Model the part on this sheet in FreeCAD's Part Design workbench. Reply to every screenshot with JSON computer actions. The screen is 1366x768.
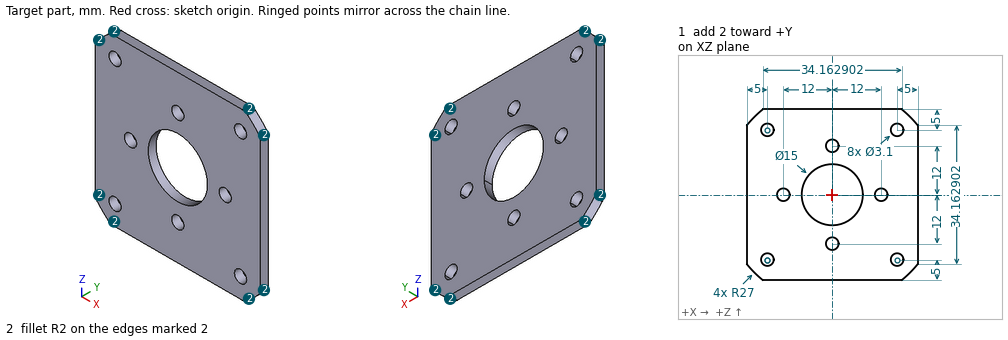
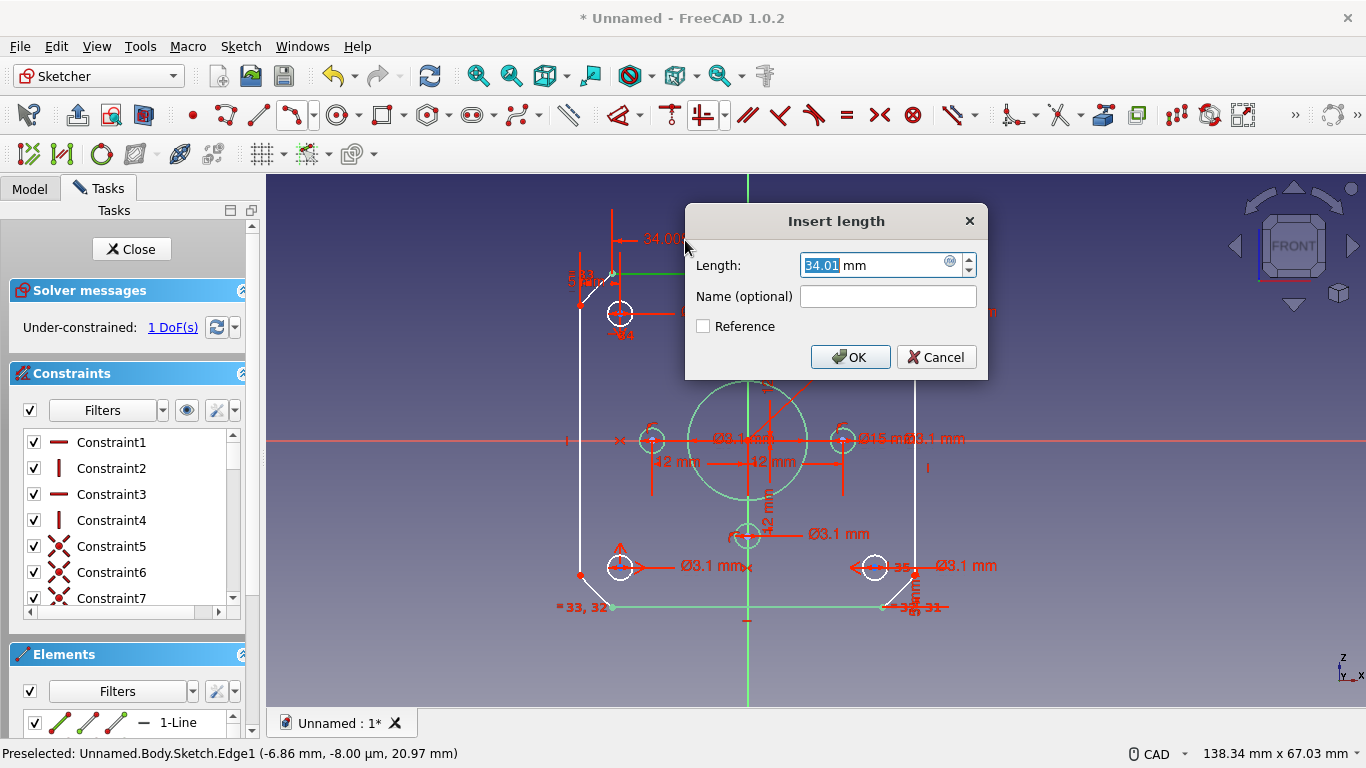
{"action": "type", "text": "34.162902"}
{"action": "key", "text": "Return"}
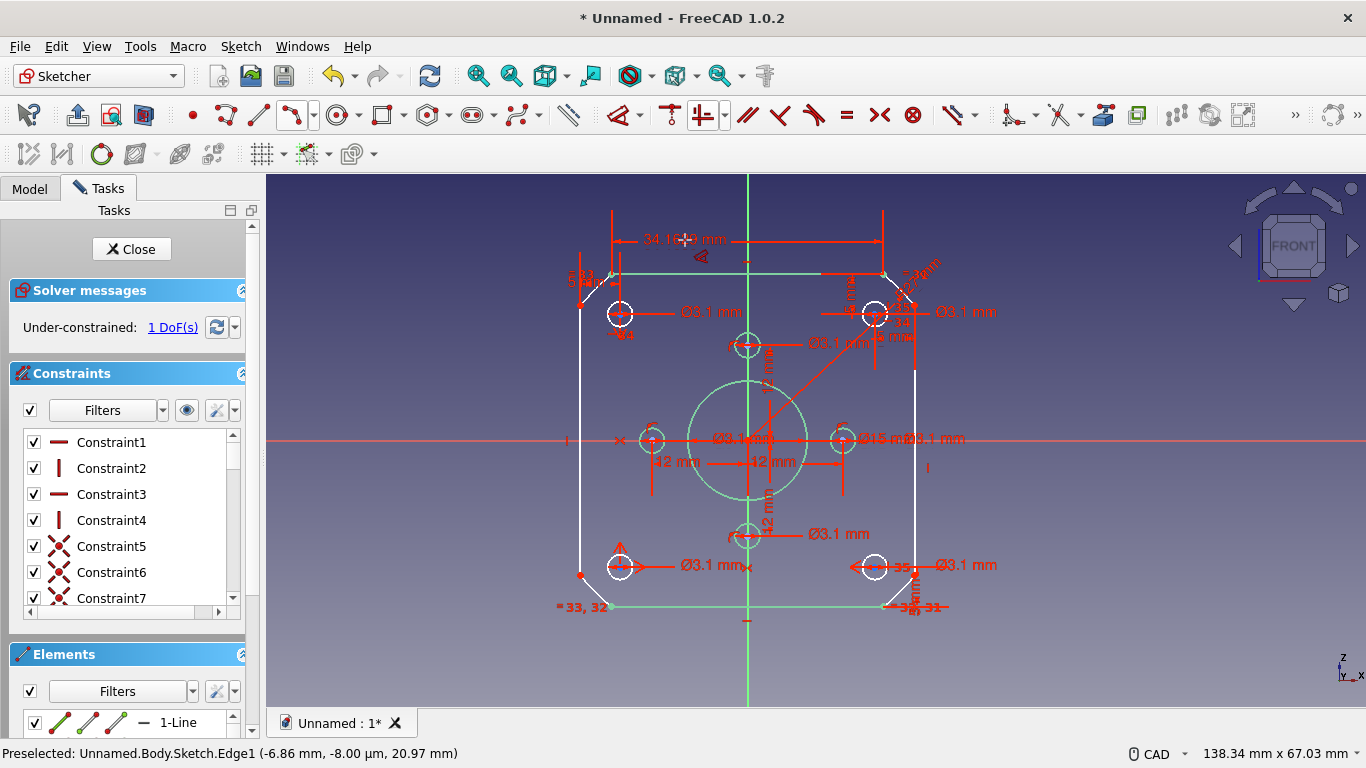
{"action": "left_click", "coordinate": [915, 387]}
{"action": "left_click", "coordinate": [949, 379]}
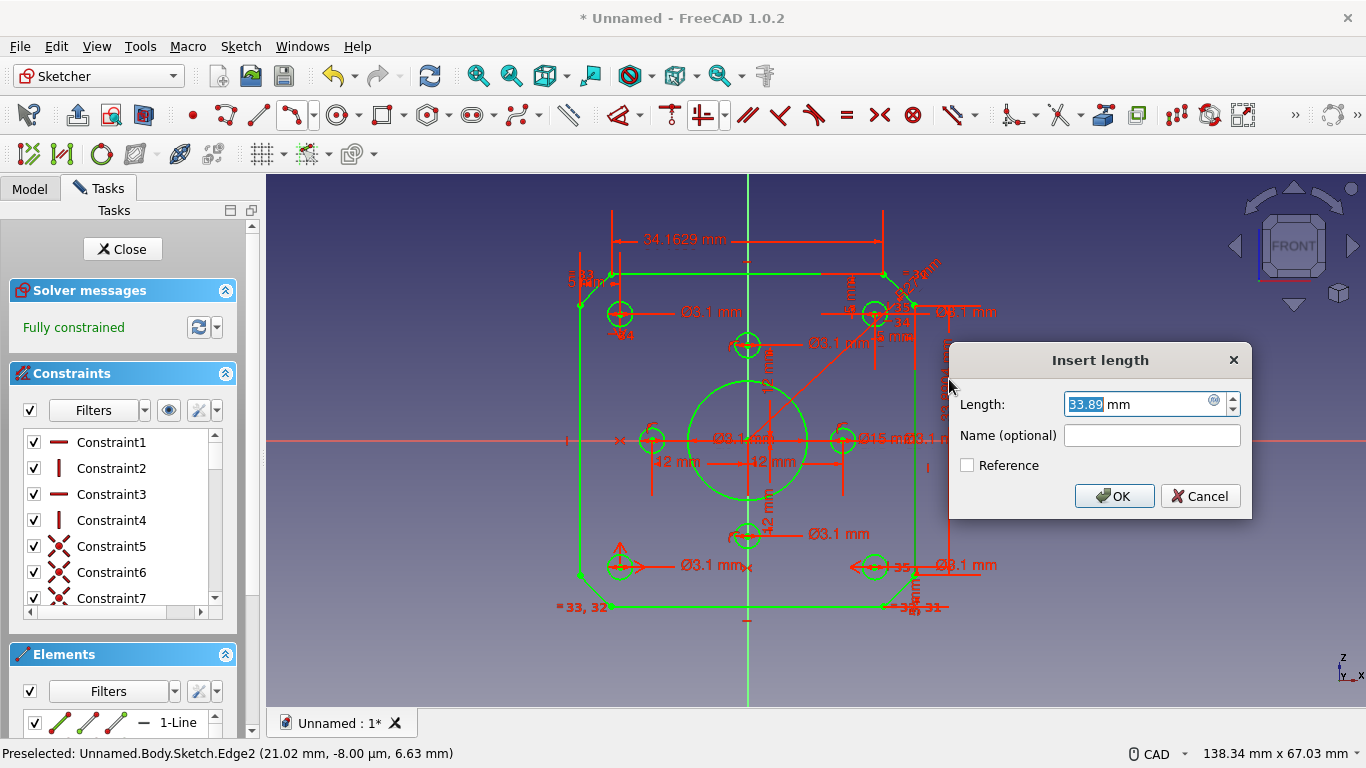
{"action": "type", "text": "34.162902"}
{"action": "key", "text": "Return"}
{"action": "key", "text": "Escape"}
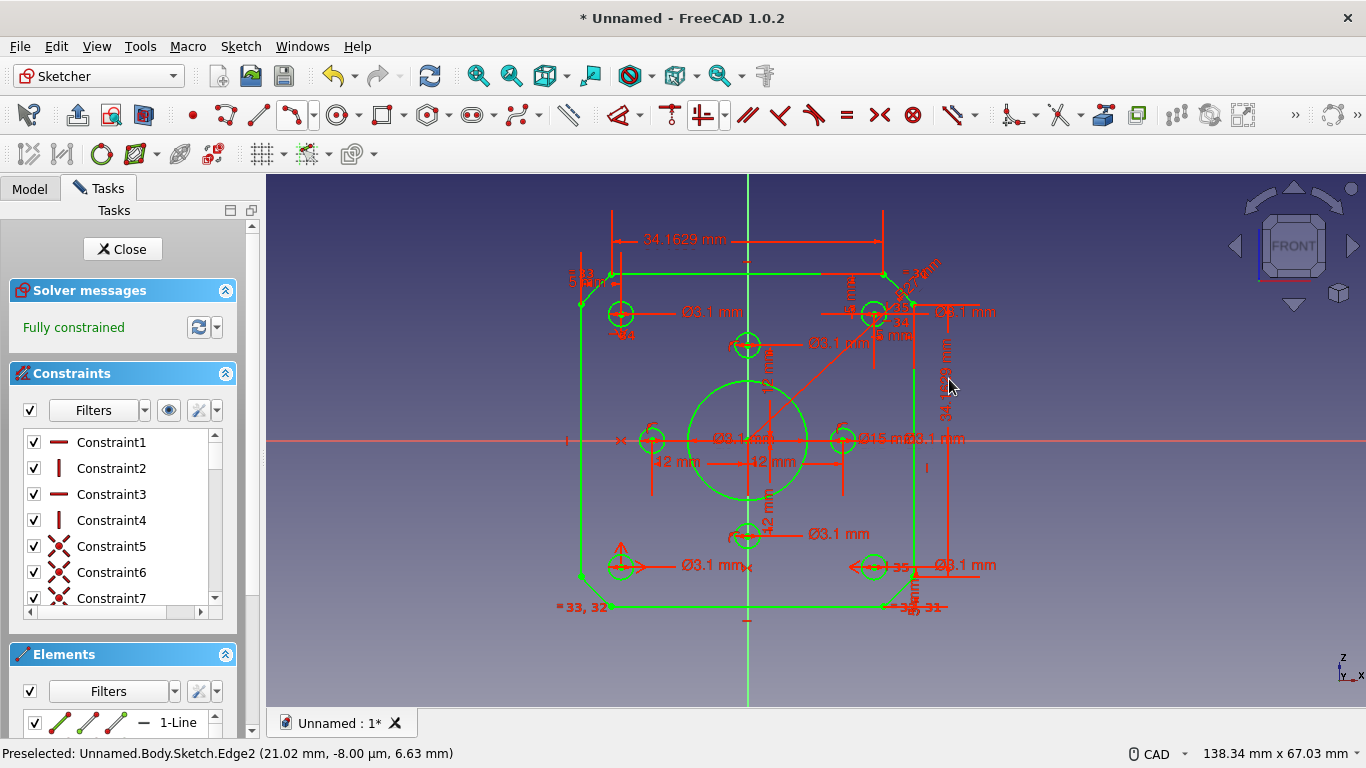
{"action": "left_click", "coordinate": [123, 249]}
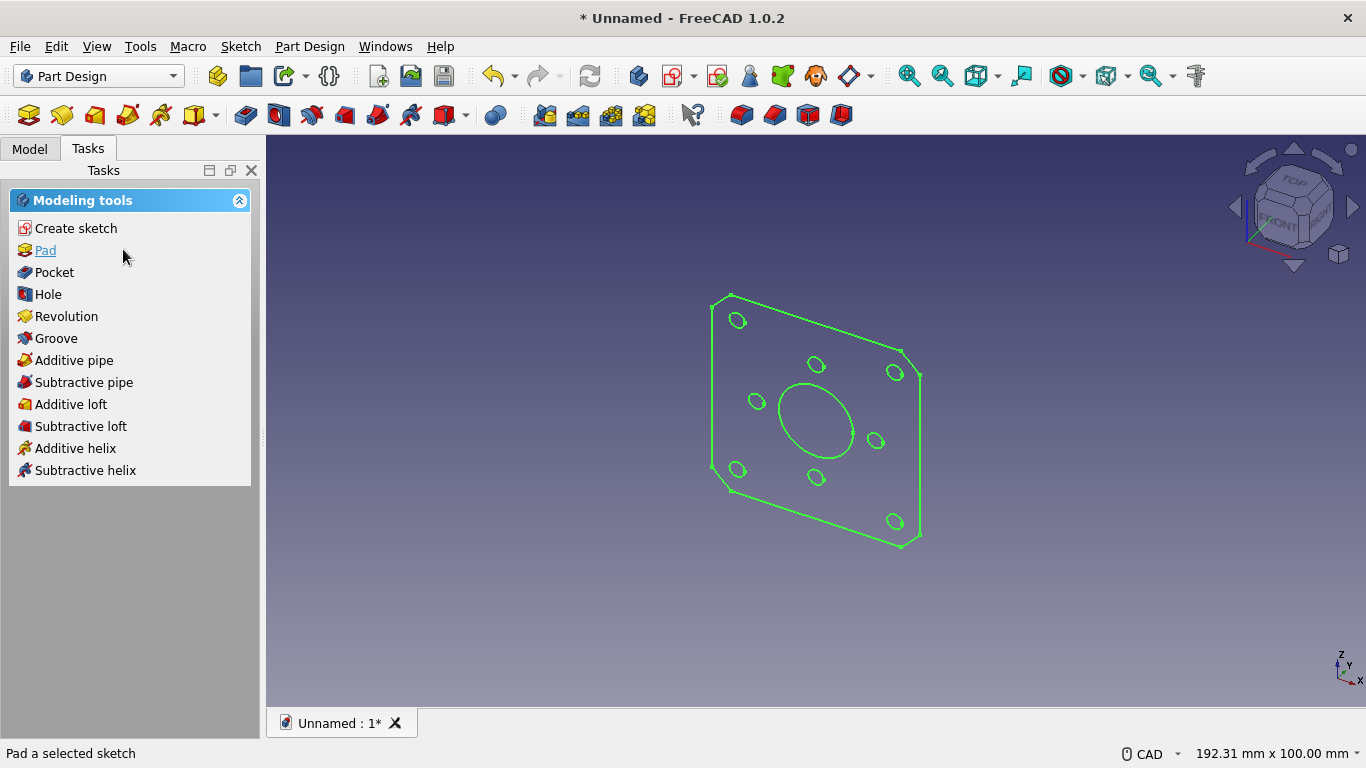
{"action": "left_click", "coordinate": [29, 116]}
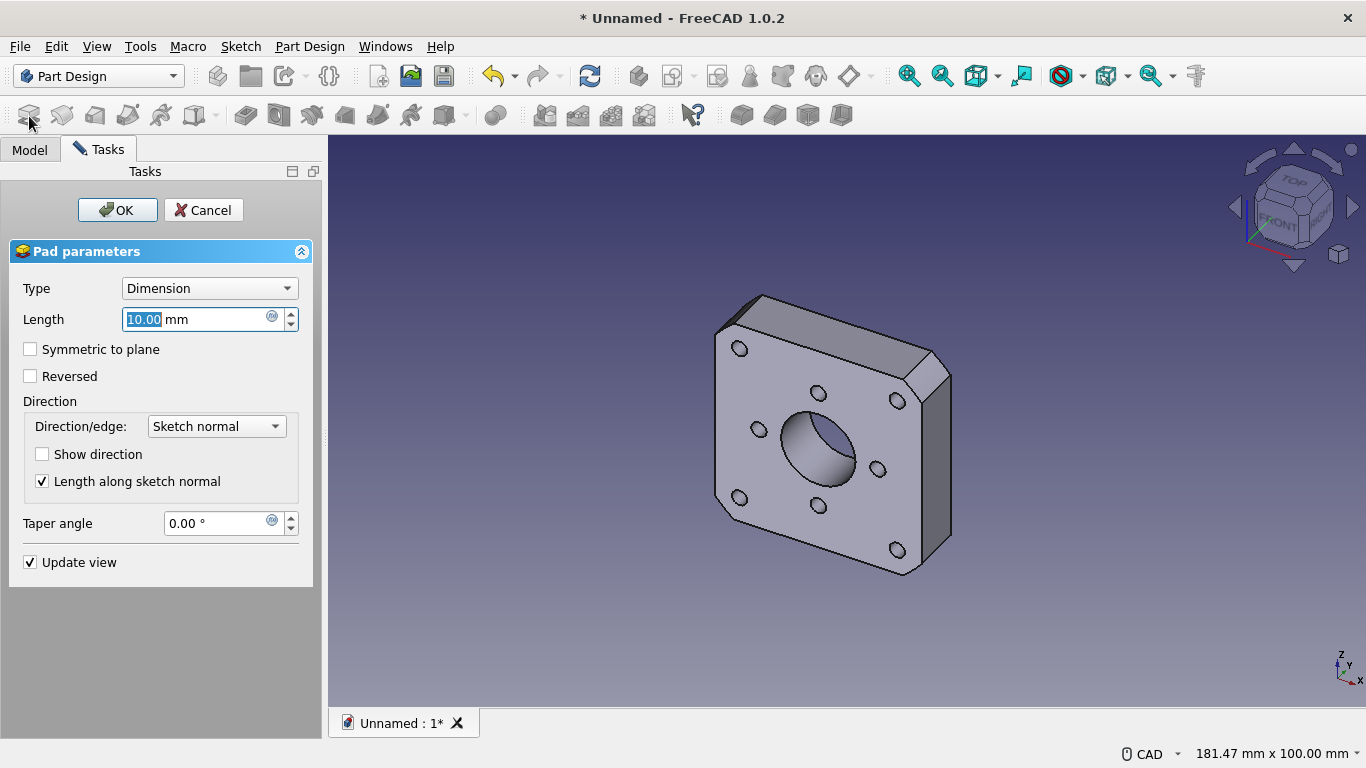
{"action": "type", "text": "2"}
{"action": "key", "text": "Tab"}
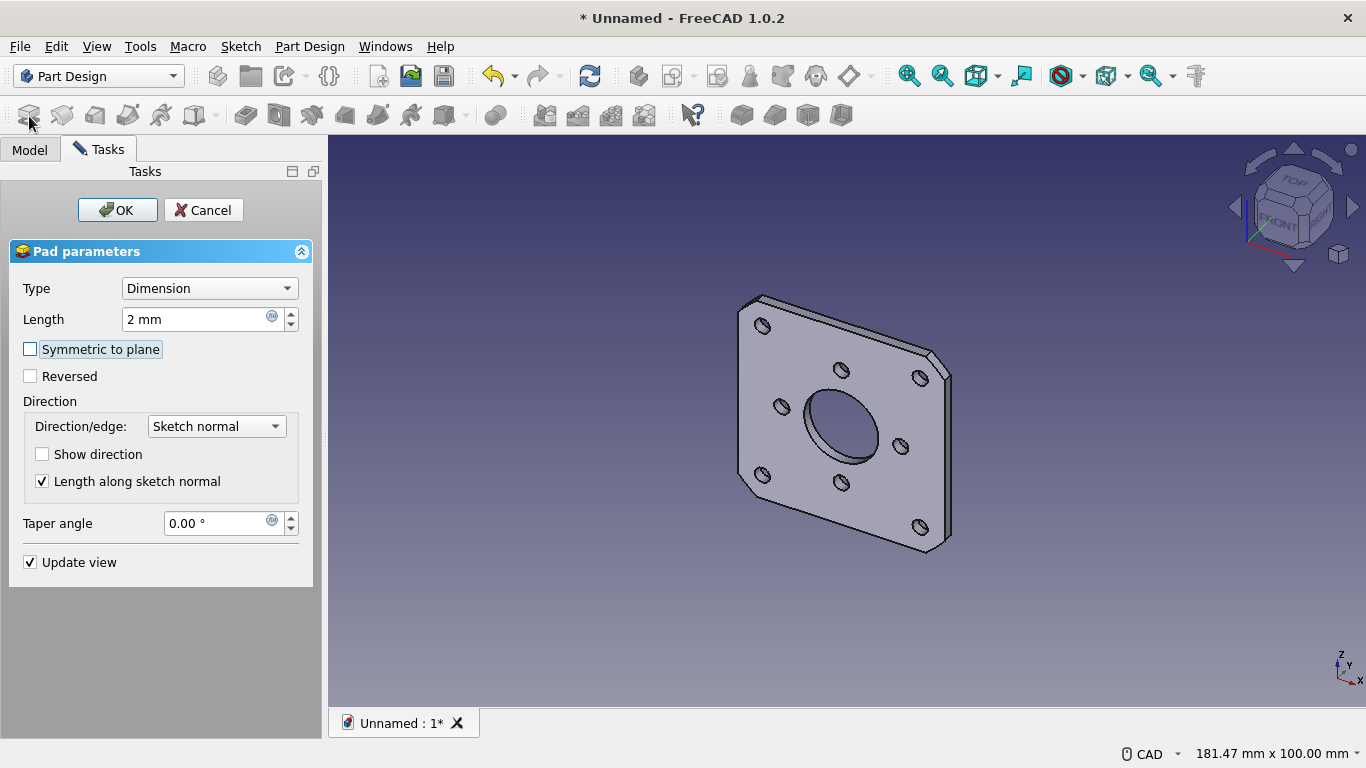
{"action": "left_click", "coordinate": [31, 376]}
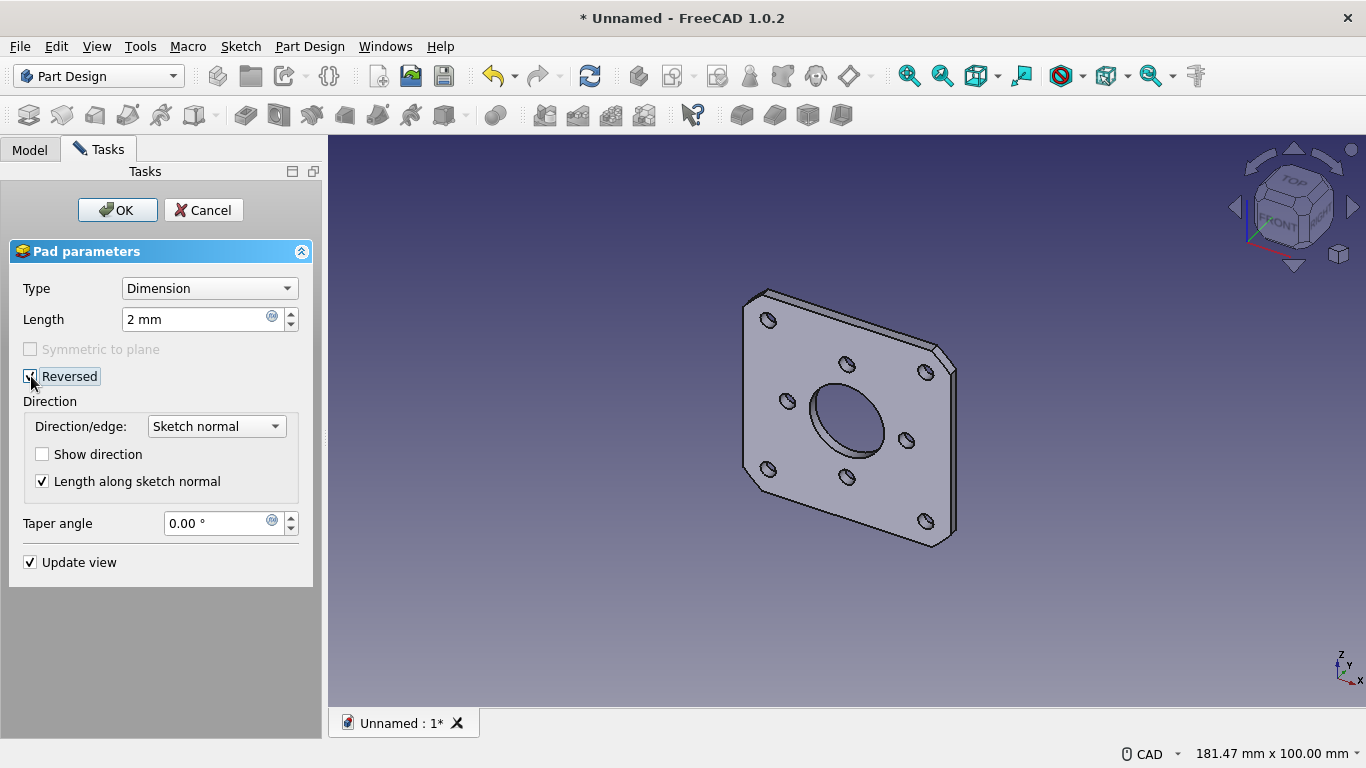
{"action": "left_click", "coordinate": [118, 210]}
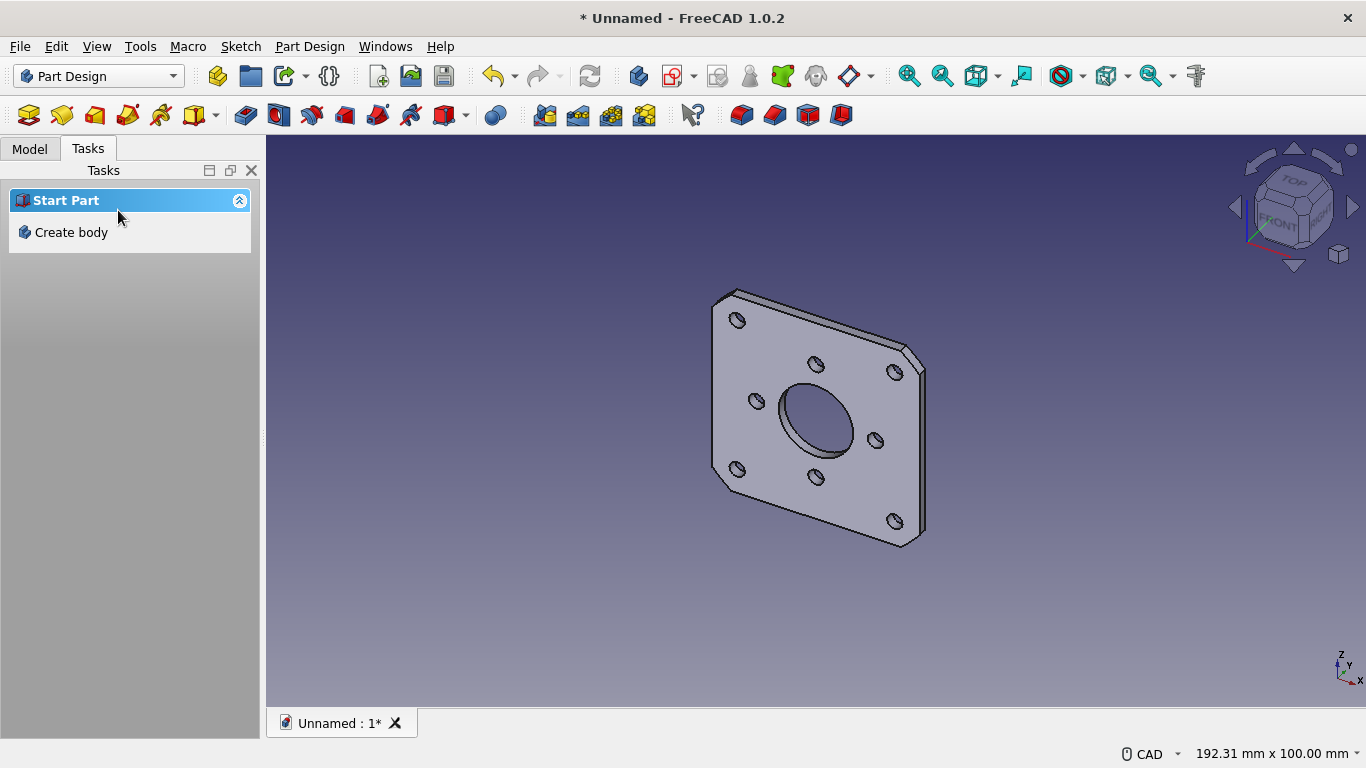
{"action": "scroll", "coordinate": [903, 347], "scroll_direction": "up", "scroll_amount": 7}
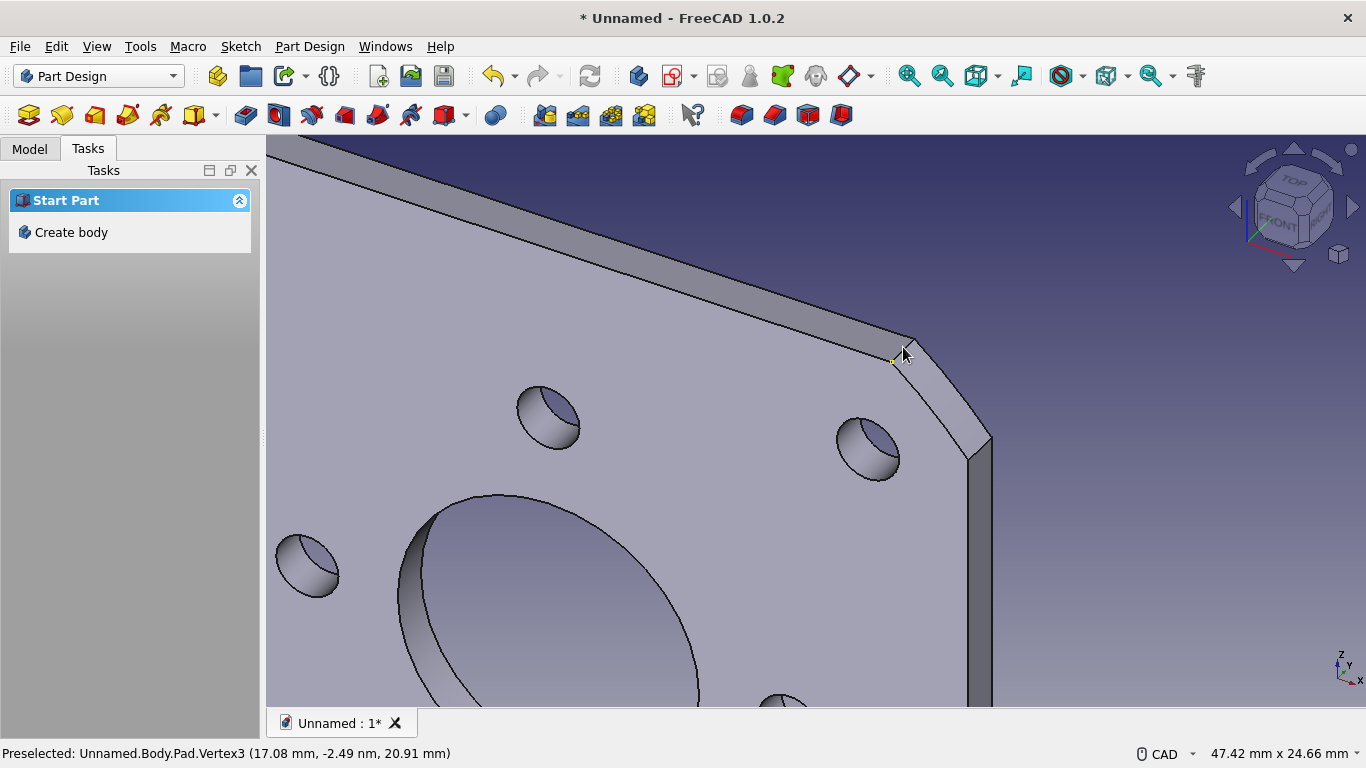
{"action": "left_click", "coordinate": [903, 350]}